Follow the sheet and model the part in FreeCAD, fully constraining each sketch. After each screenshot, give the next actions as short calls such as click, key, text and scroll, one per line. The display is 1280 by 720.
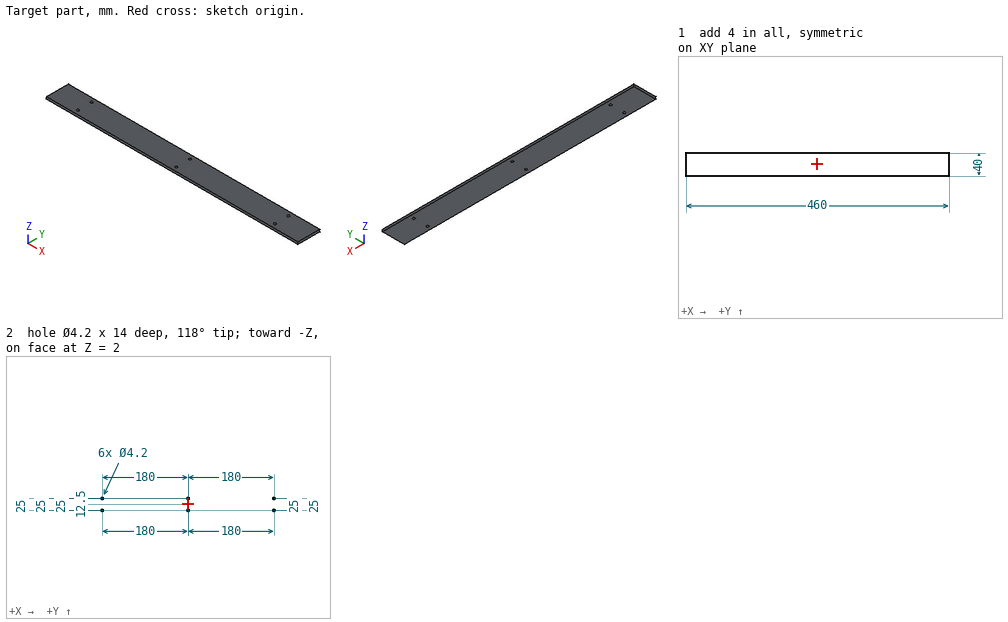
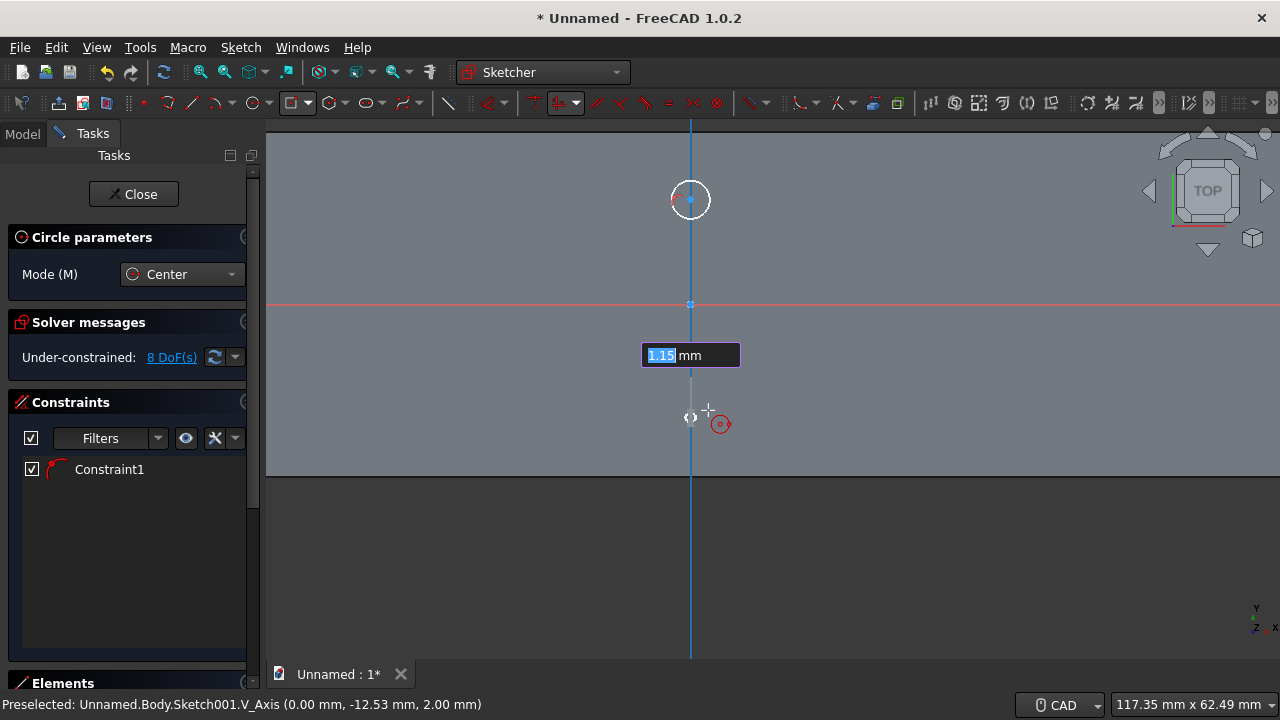
click(708, 406)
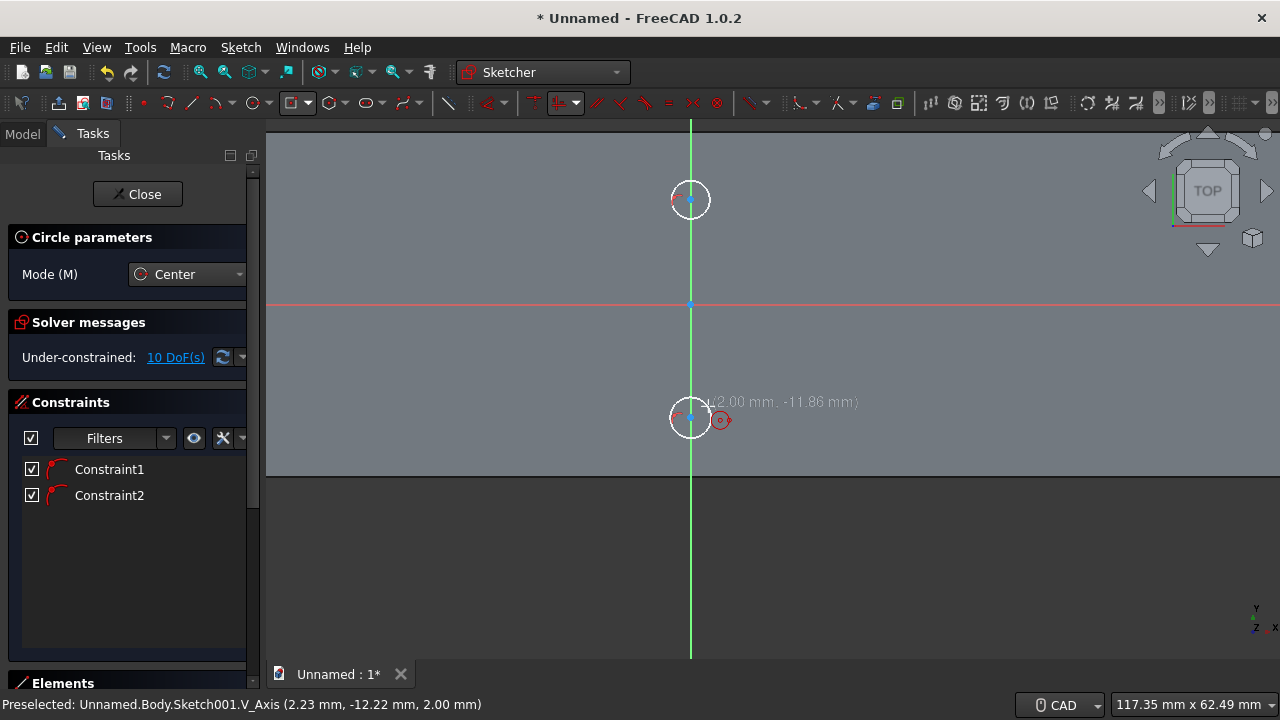
scroll(708, 410, down, 8)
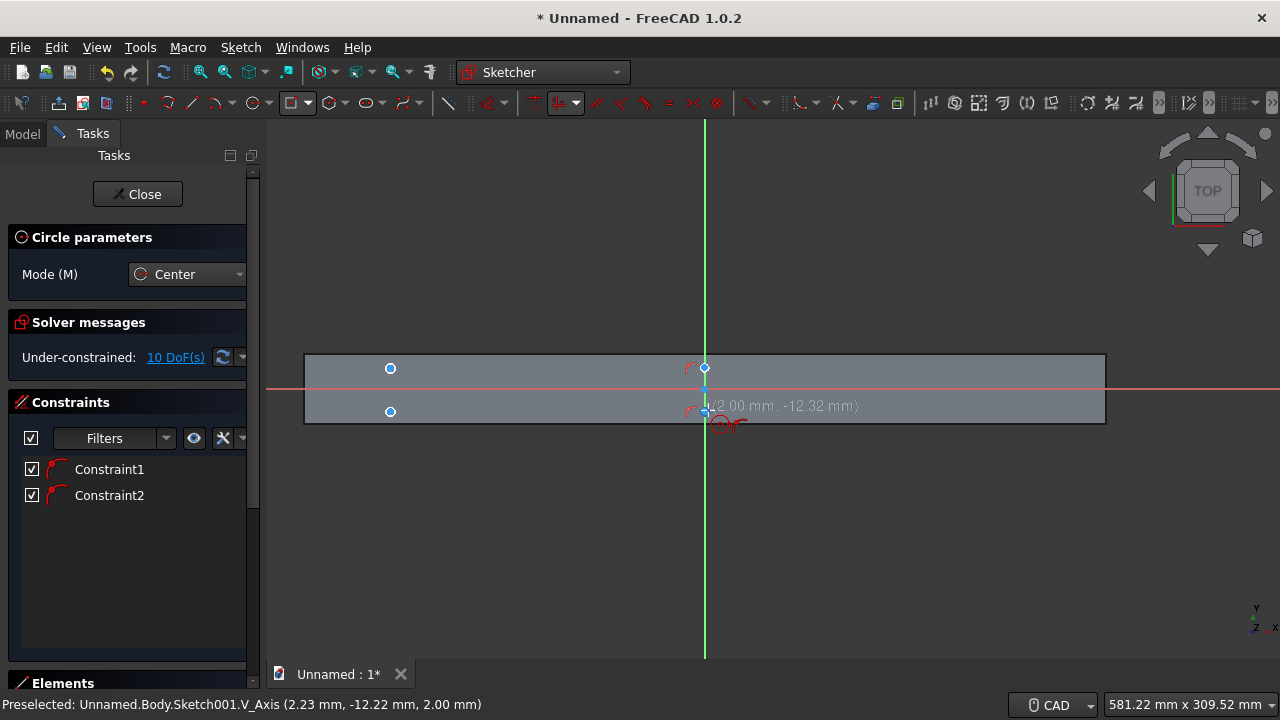
scroll(1019, 367, up, 10)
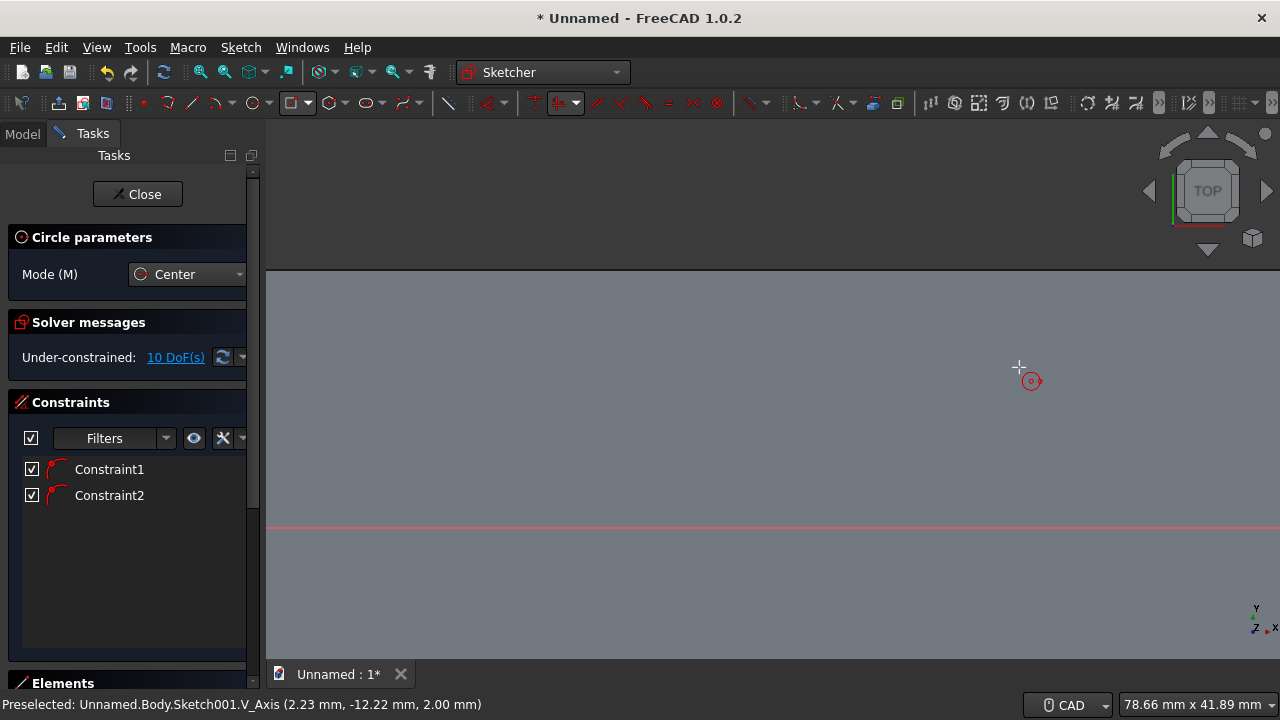
scroll(1019, 367, down, 10)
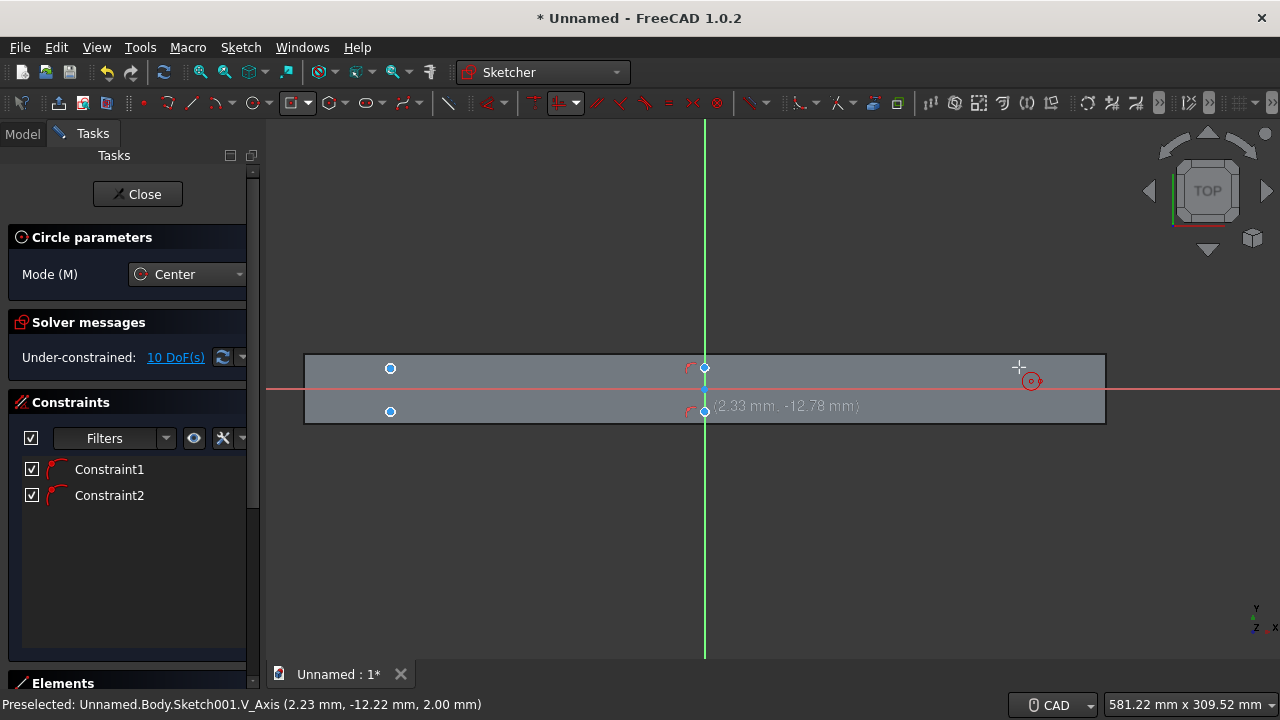
click(1019, 367)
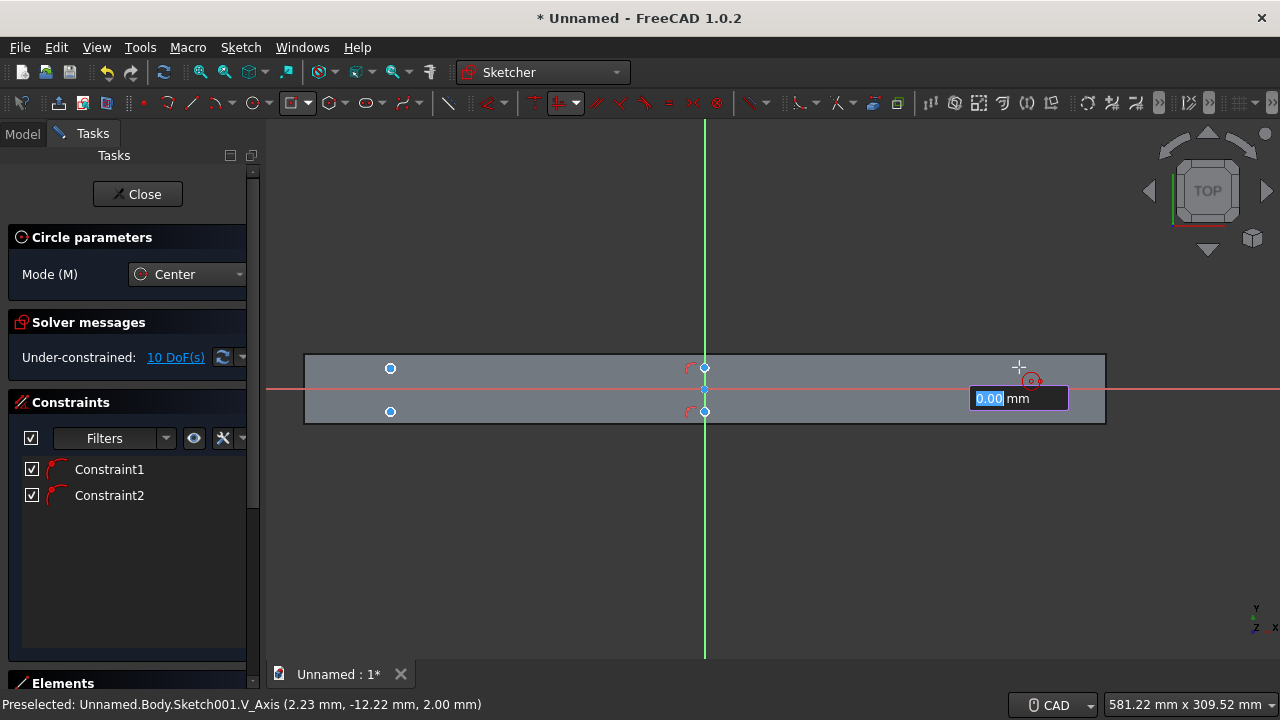
scroll(1021, 365, up, 8)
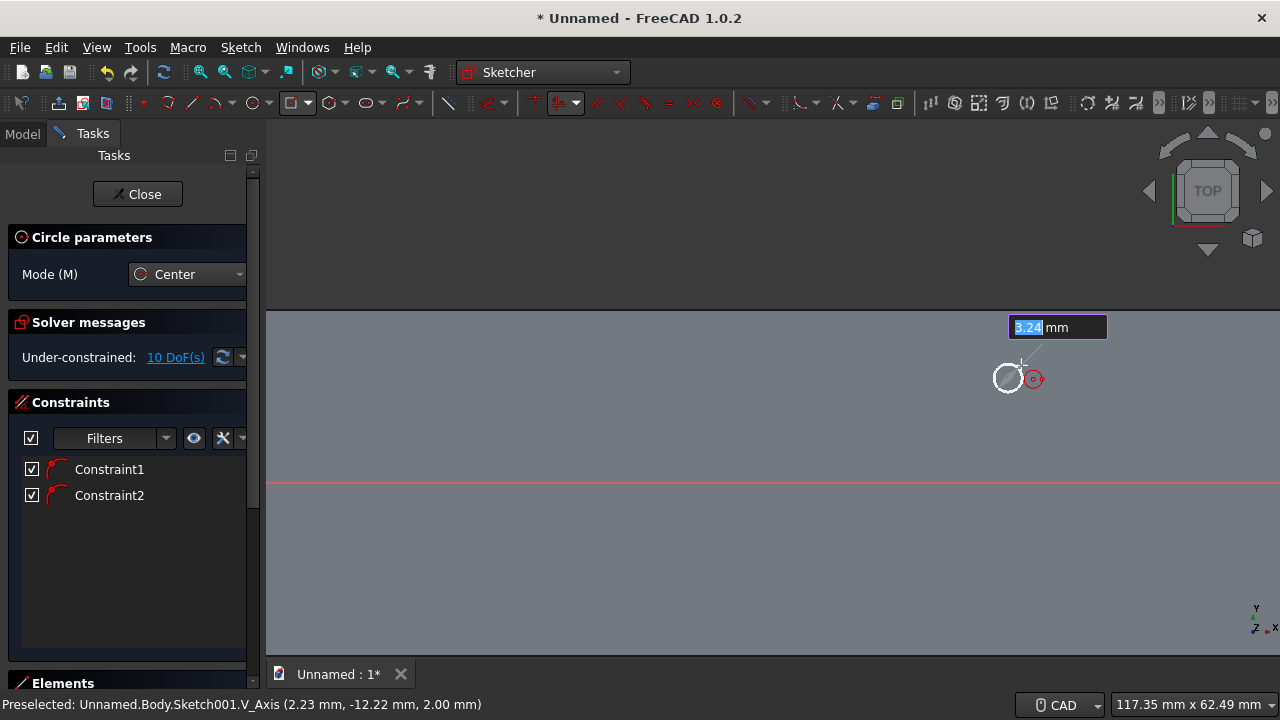
click(1020, 362)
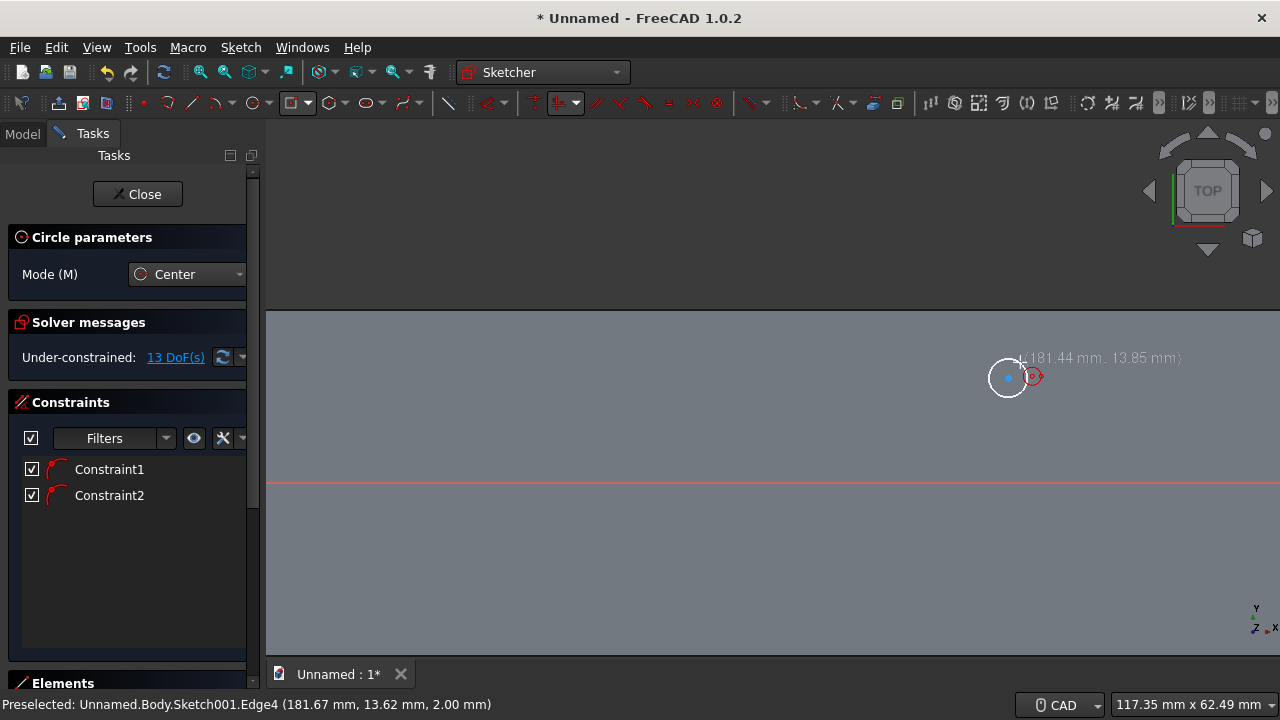
scroll(1008, 591, up, 2)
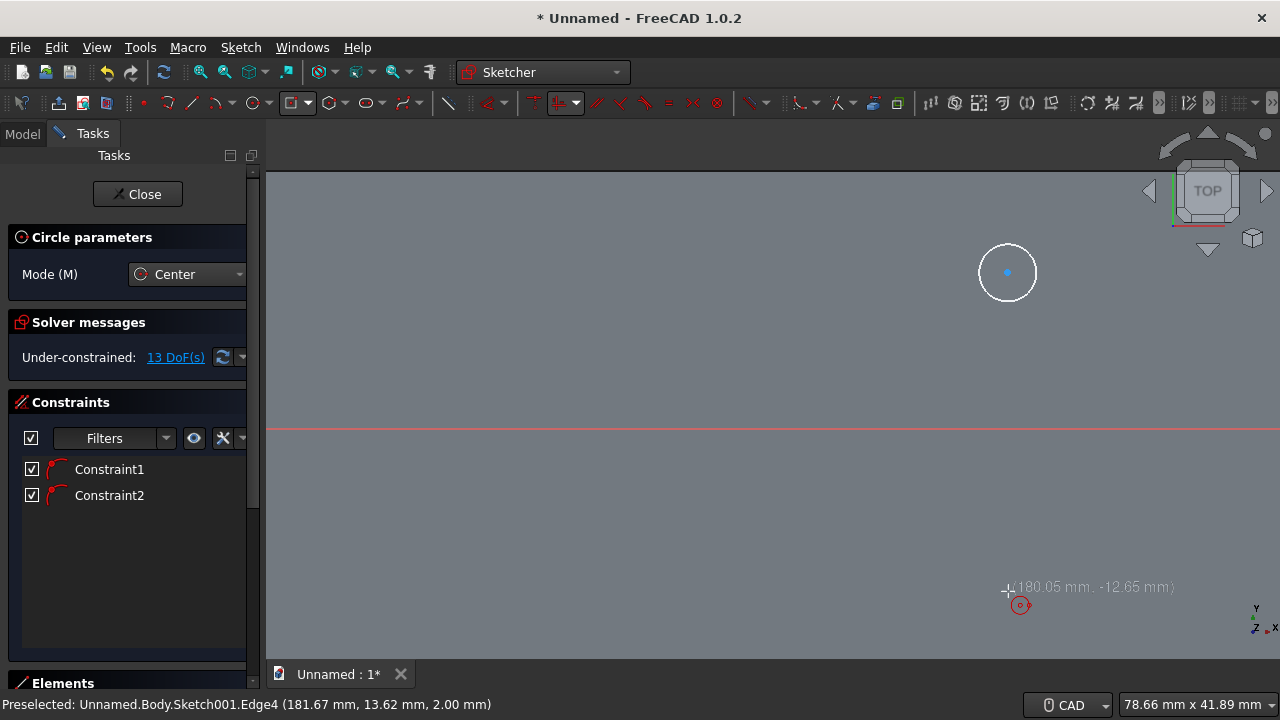
scroll(1020, 383, down, 10)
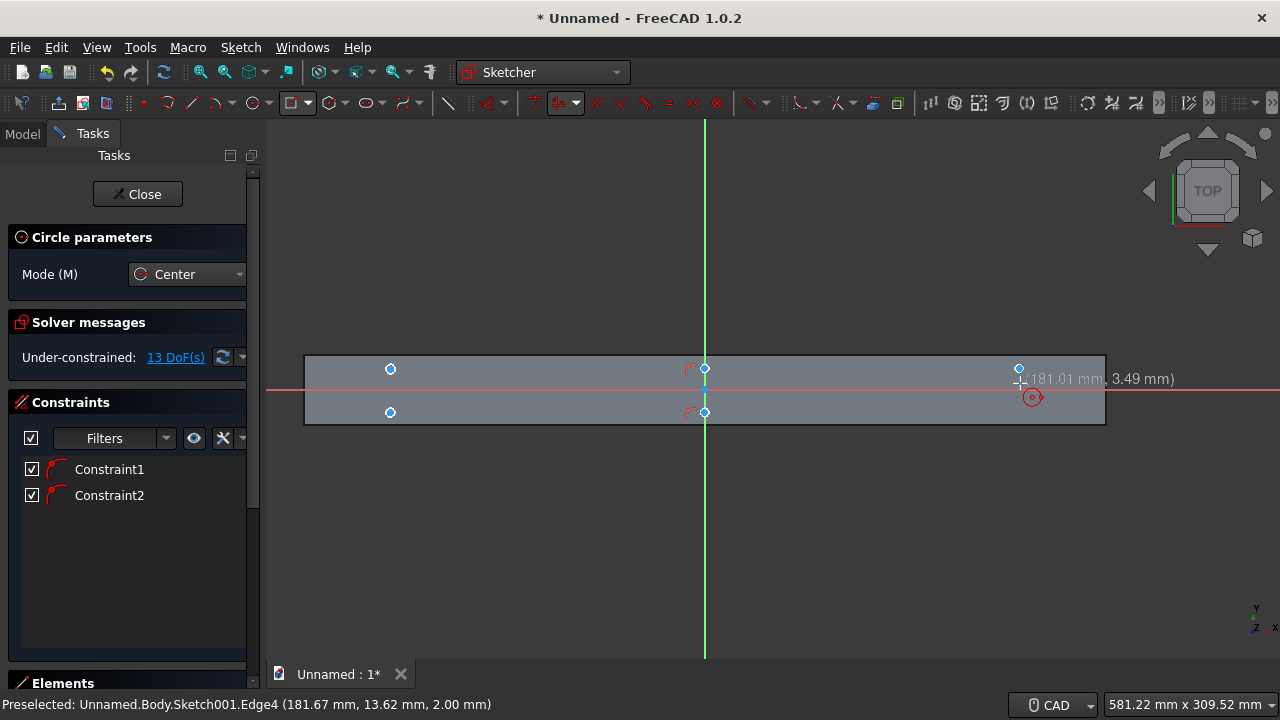
click(1019, 411)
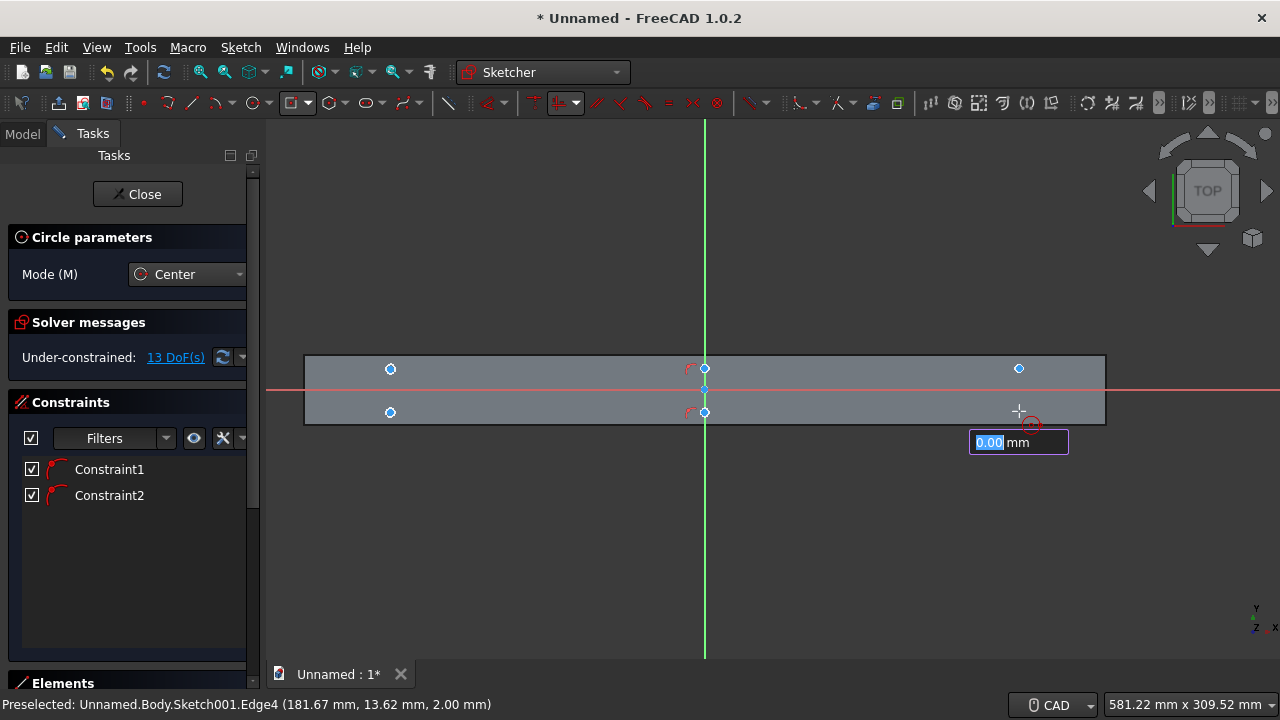
scroll(1021, 409, up, 8)